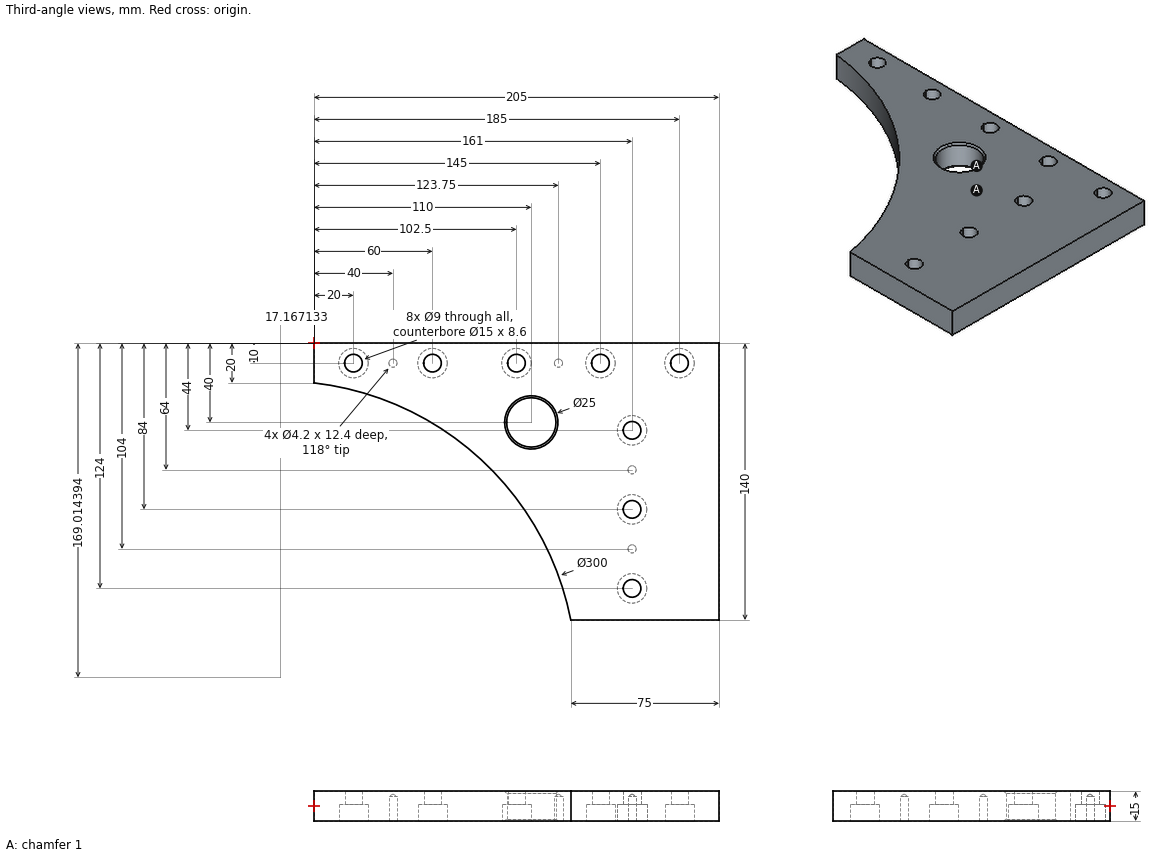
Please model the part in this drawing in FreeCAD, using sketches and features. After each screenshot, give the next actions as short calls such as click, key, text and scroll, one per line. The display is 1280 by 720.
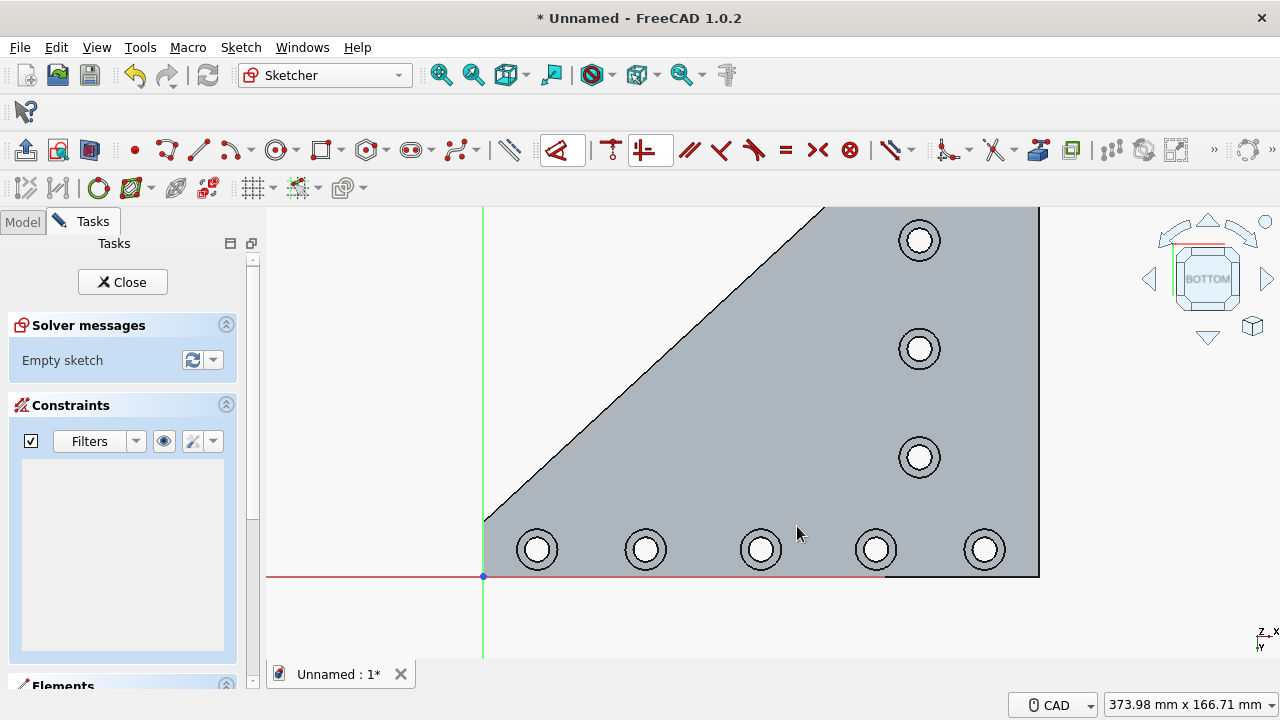
click(276, 150)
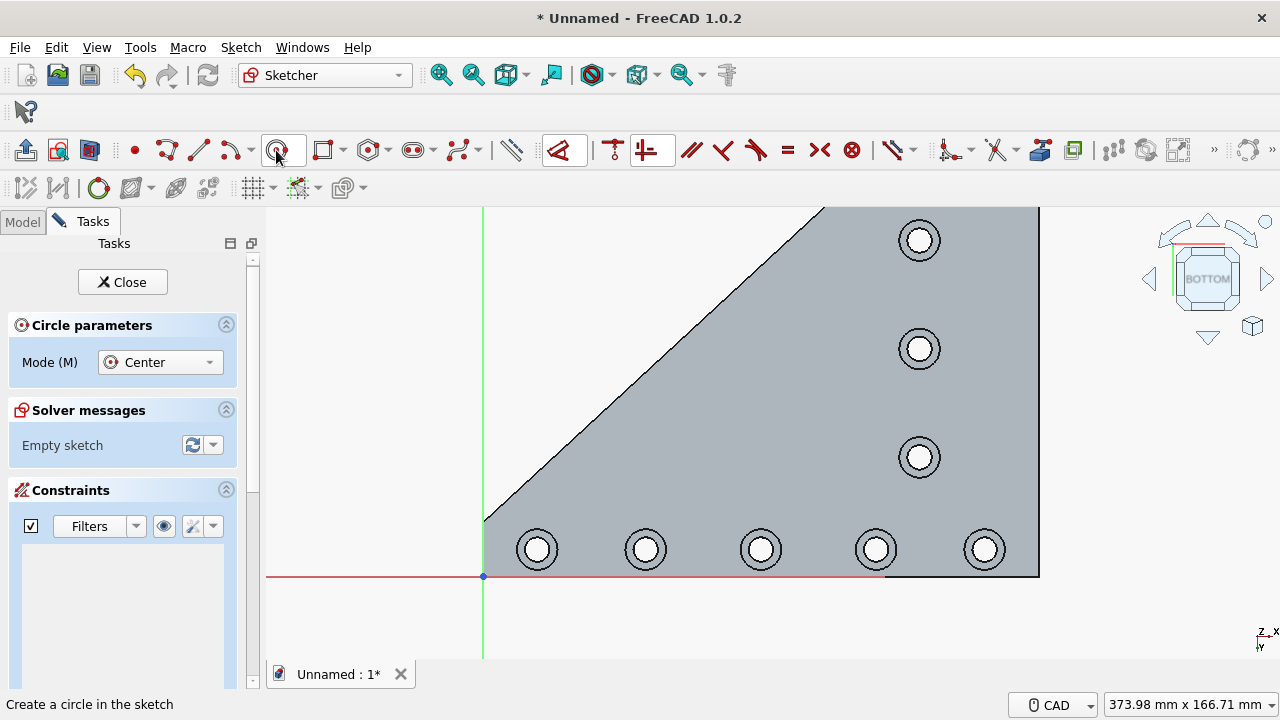
scroll(591, 550, up, 7)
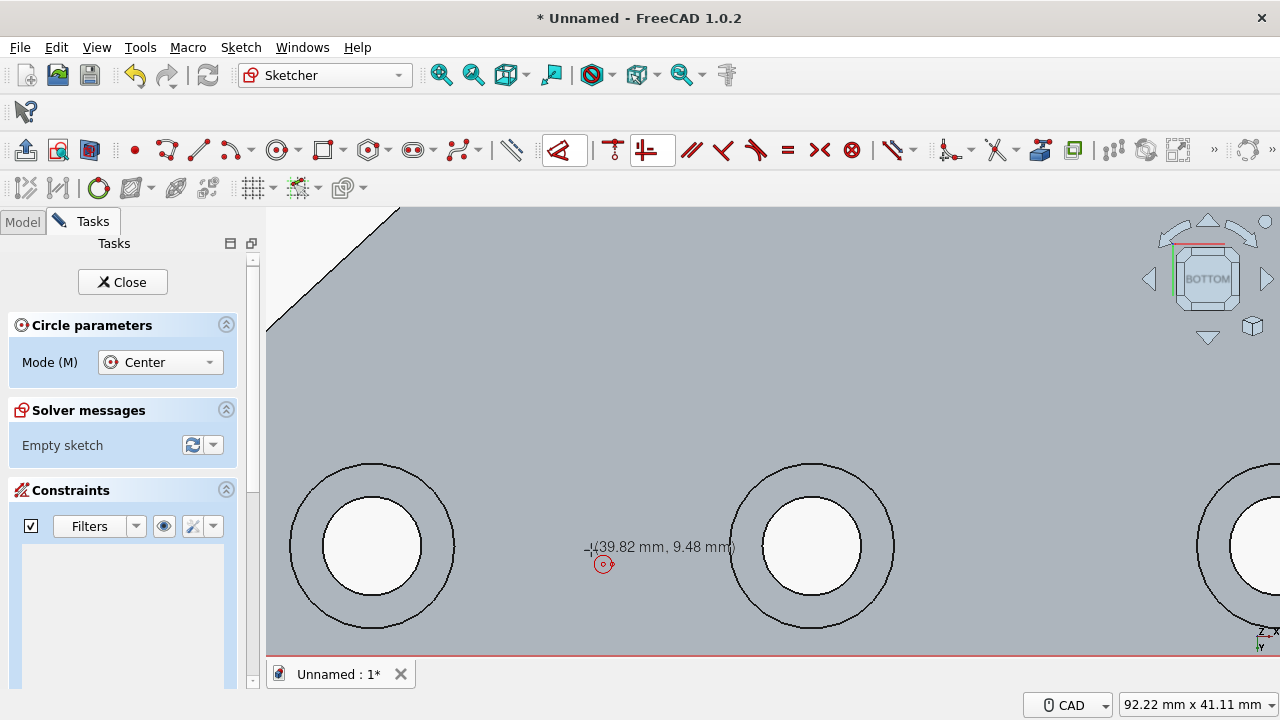
scroll(592, 551, down, 7)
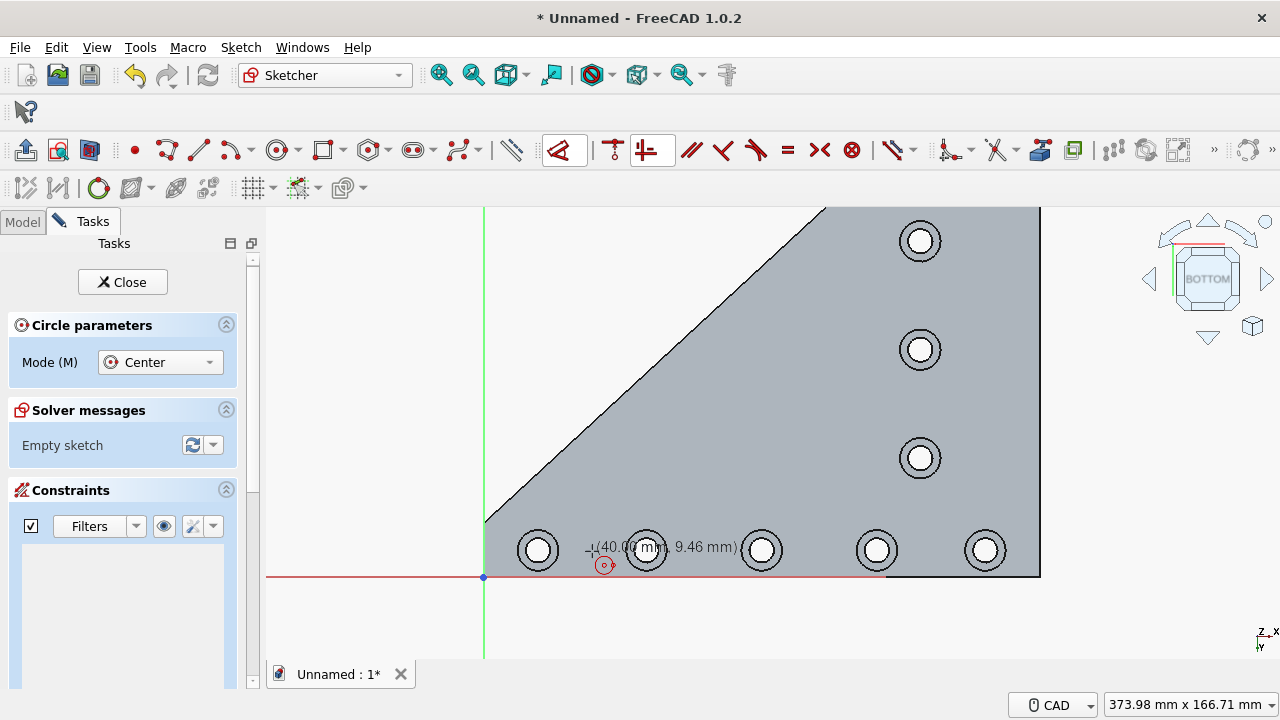
click(592, 550)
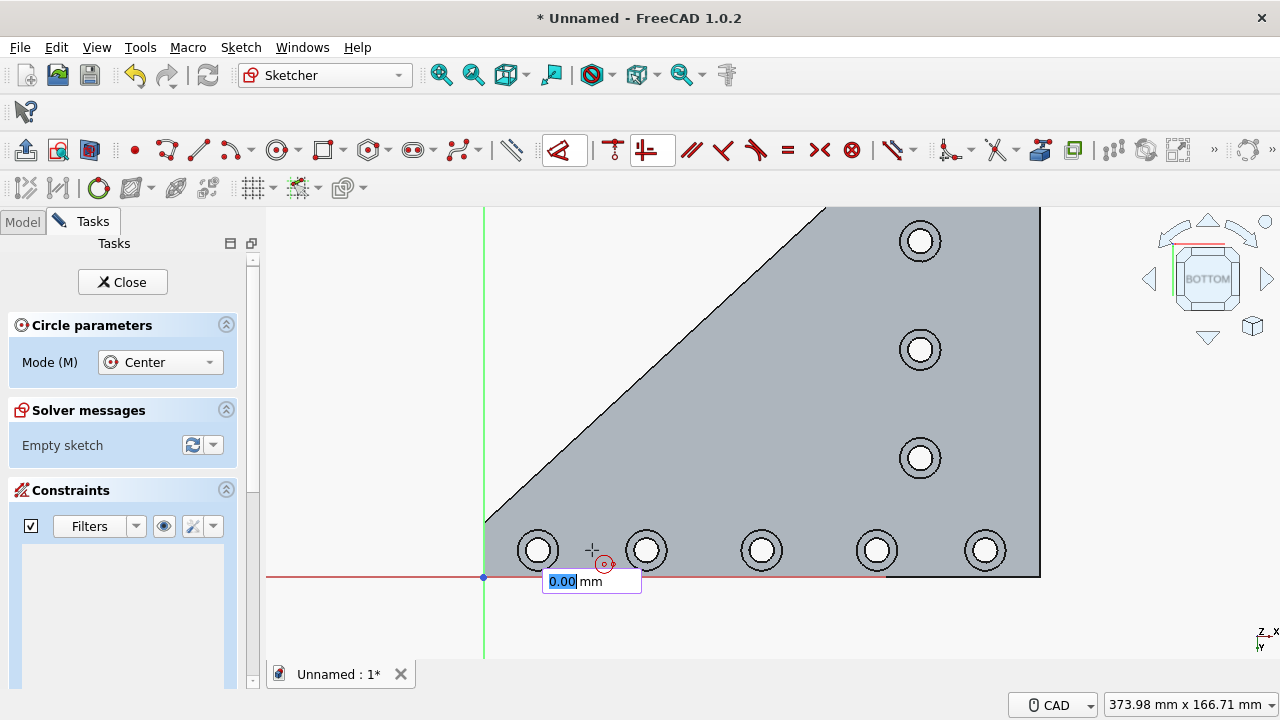
scroll(596, 546, up, 6)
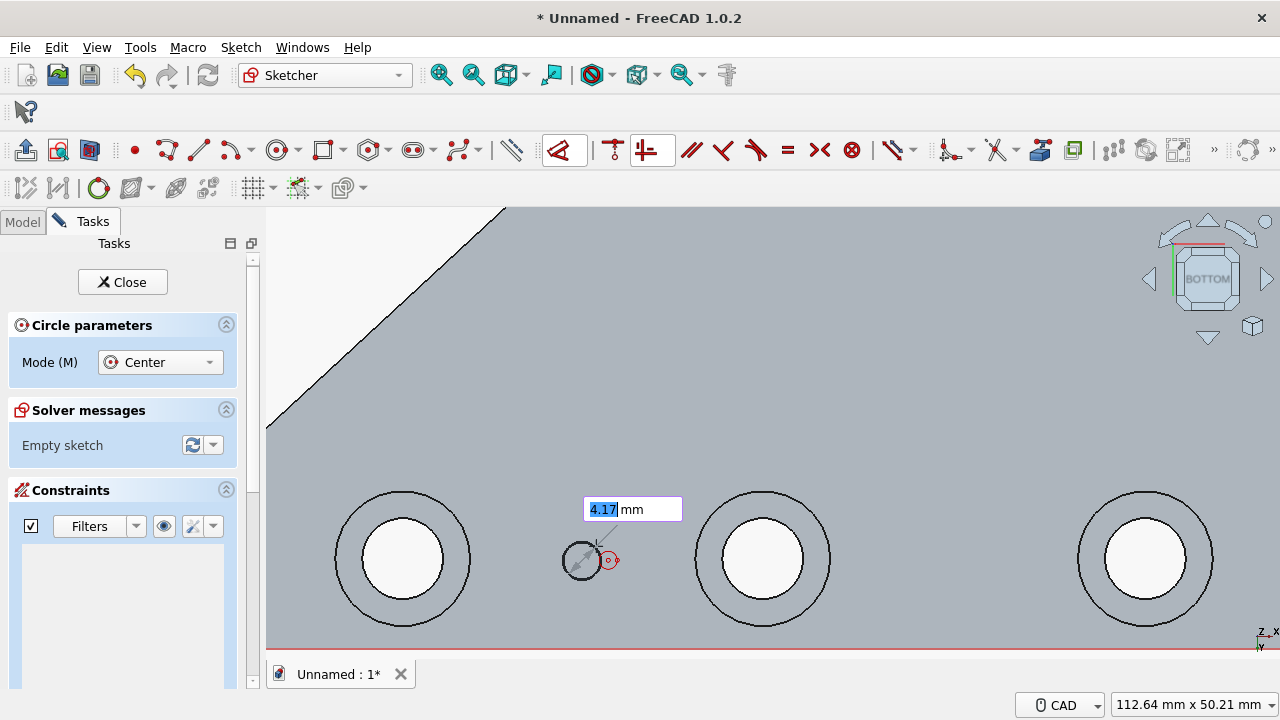
click(596, 545)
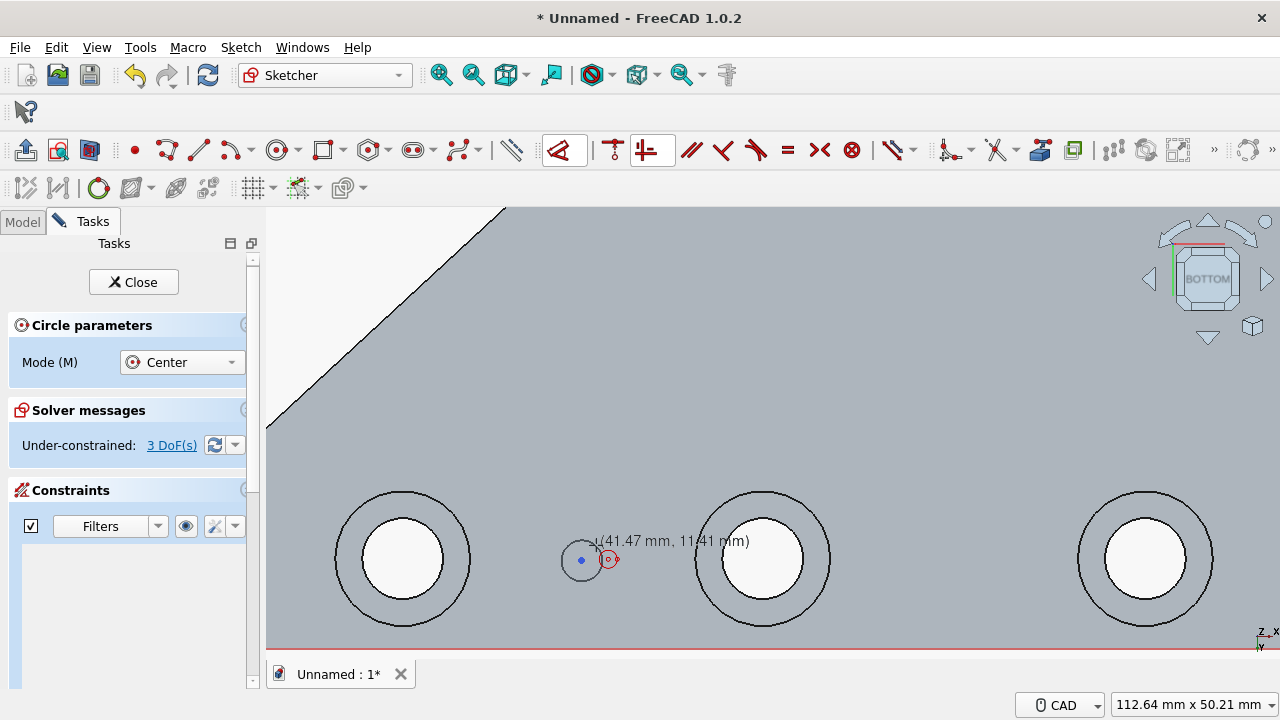
scroll(596, 546, down, 6)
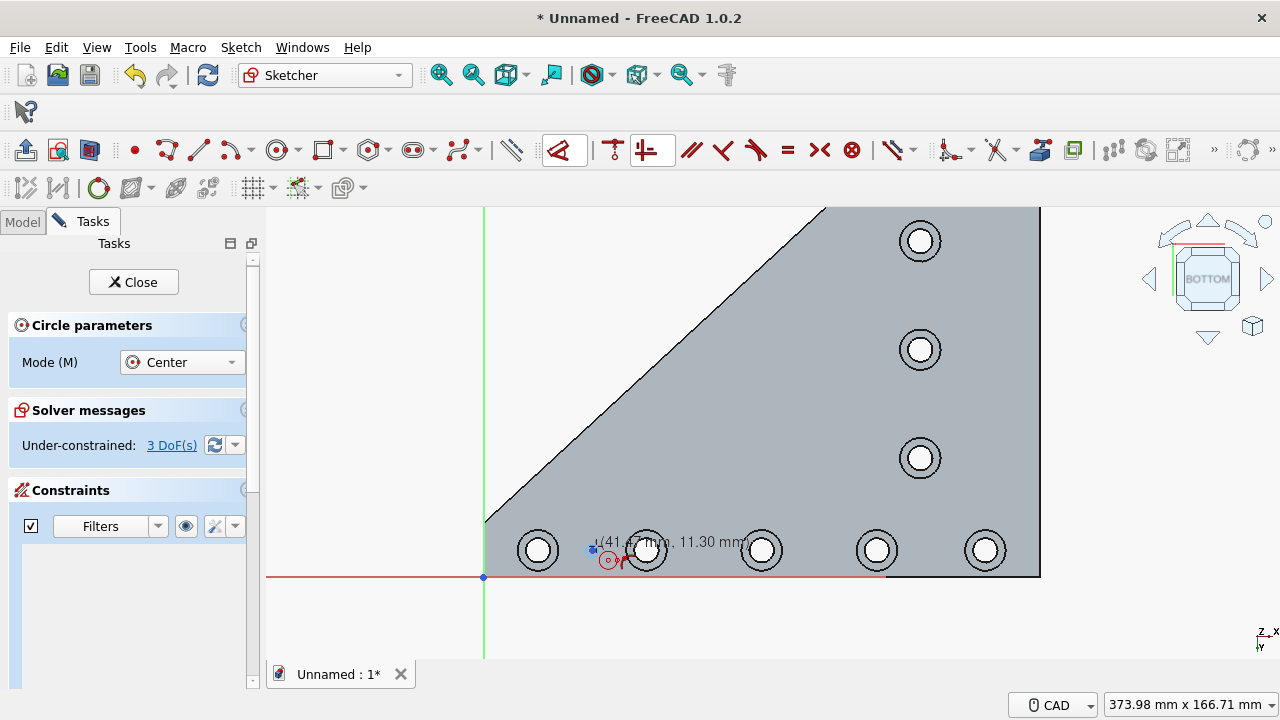
scroll(819, 550, up, 7)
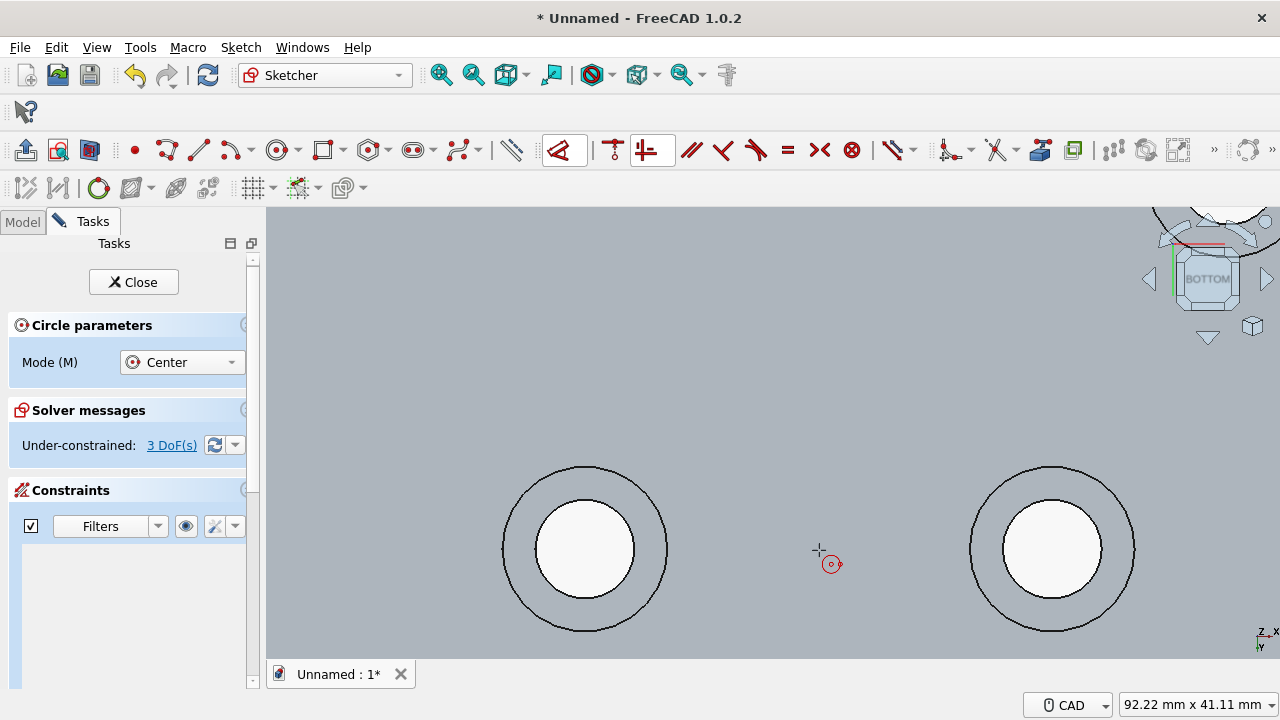
scroll(819, 550, down, 7)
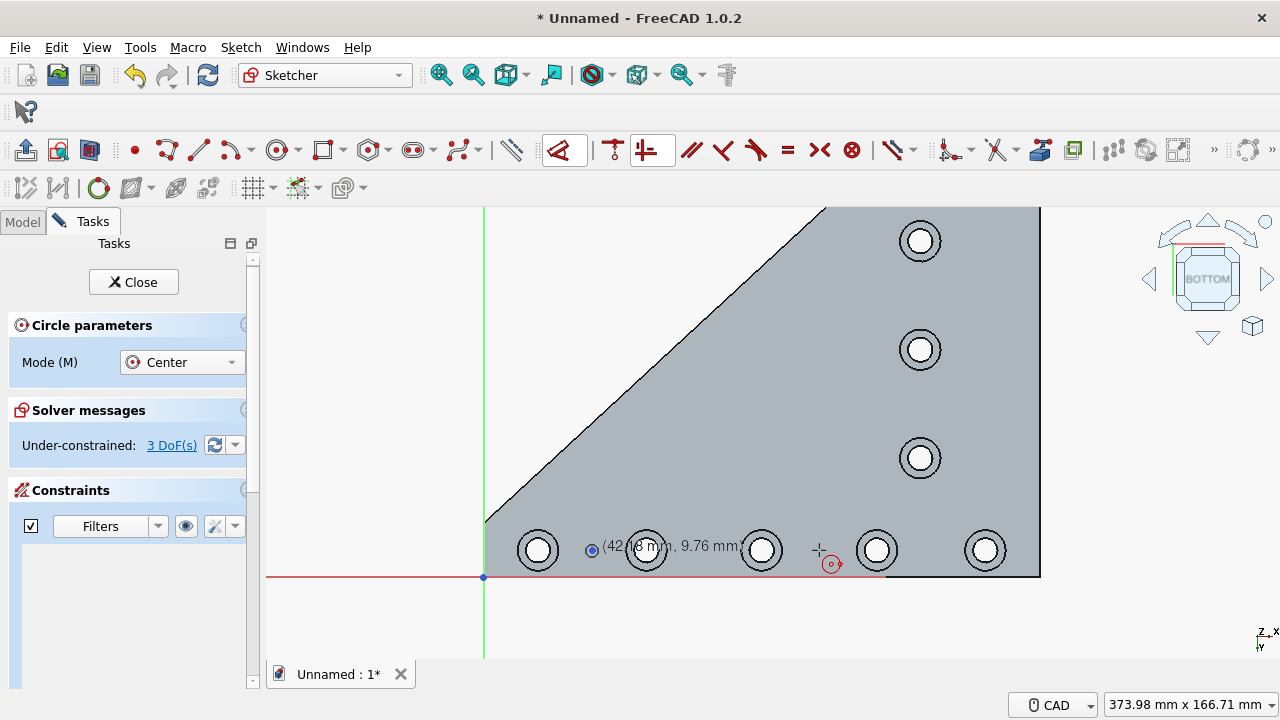
click(819, 550)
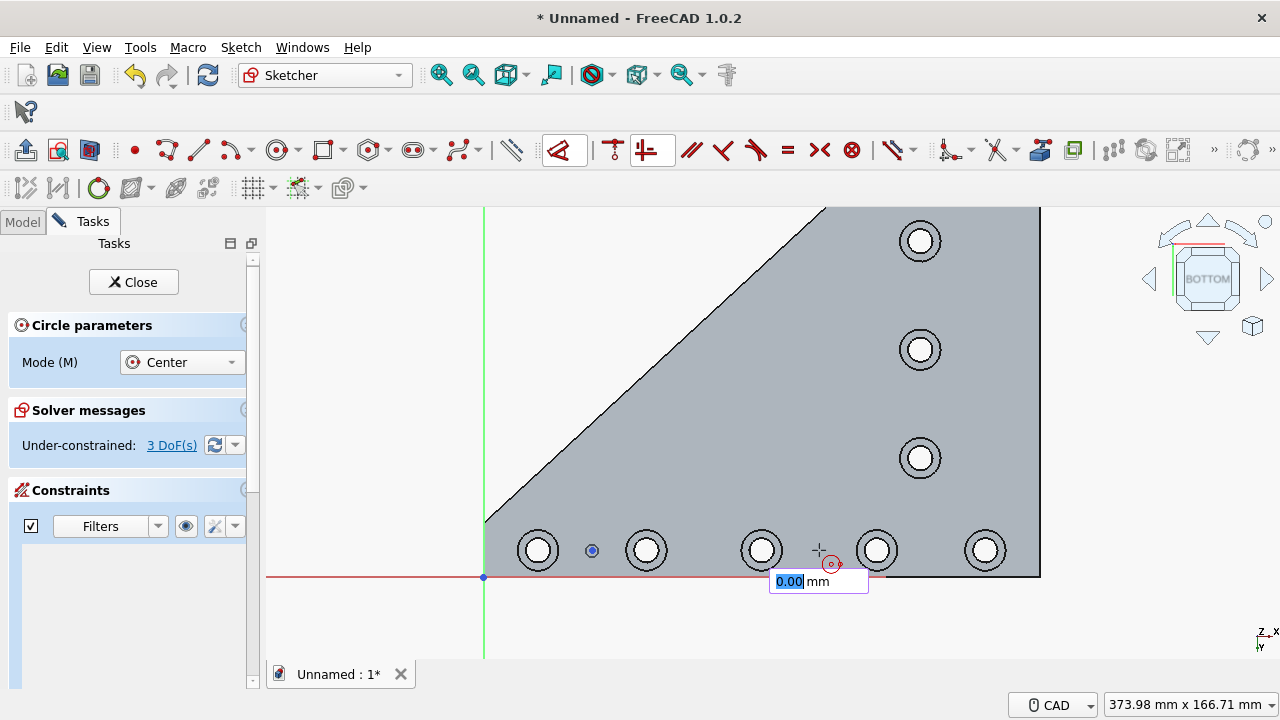
scroll(823, 546, up, 6)